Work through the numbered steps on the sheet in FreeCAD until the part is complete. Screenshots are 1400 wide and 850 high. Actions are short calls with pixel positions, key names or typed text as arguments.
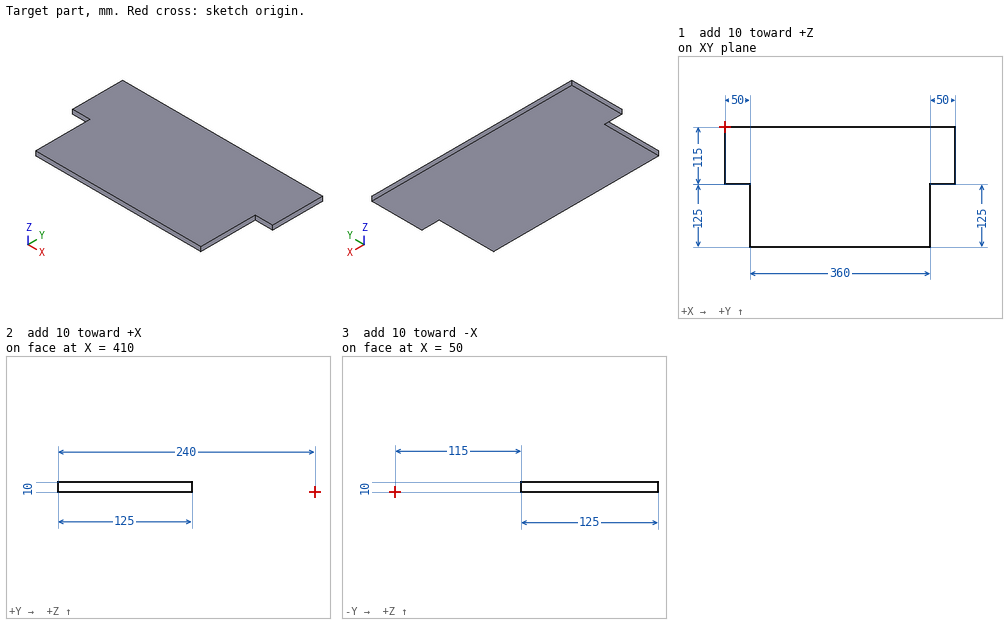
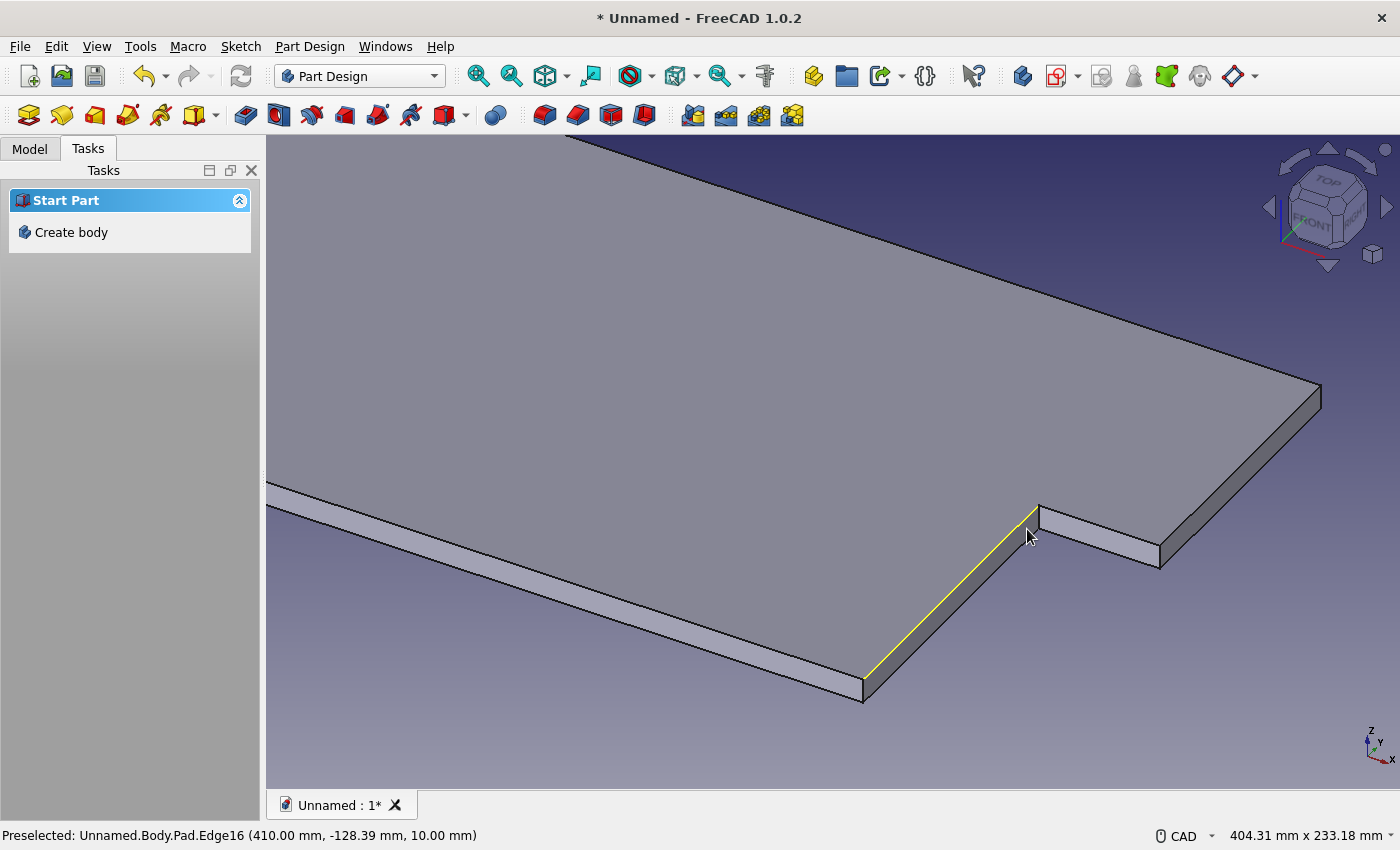
click(479, 76)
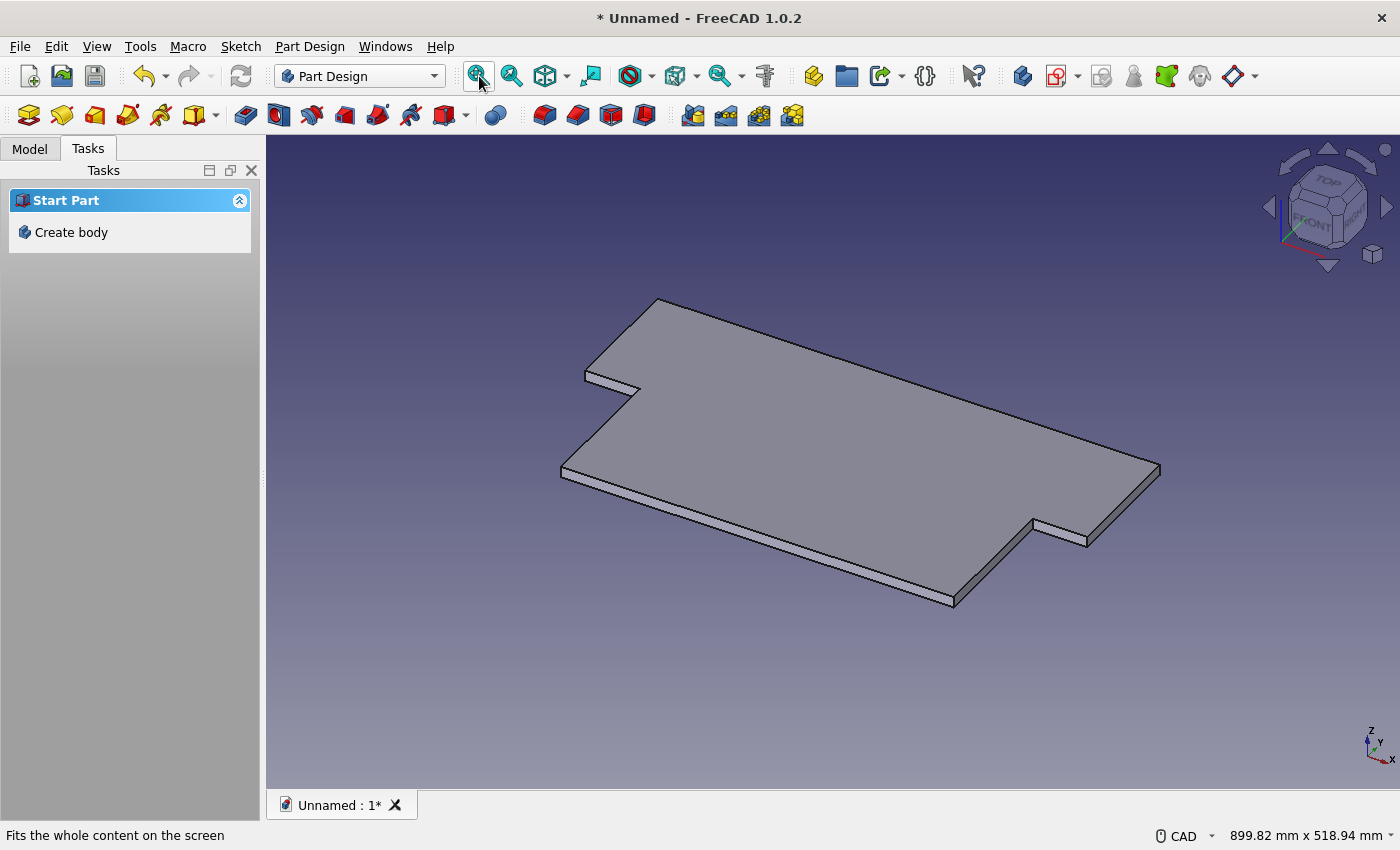
key(0)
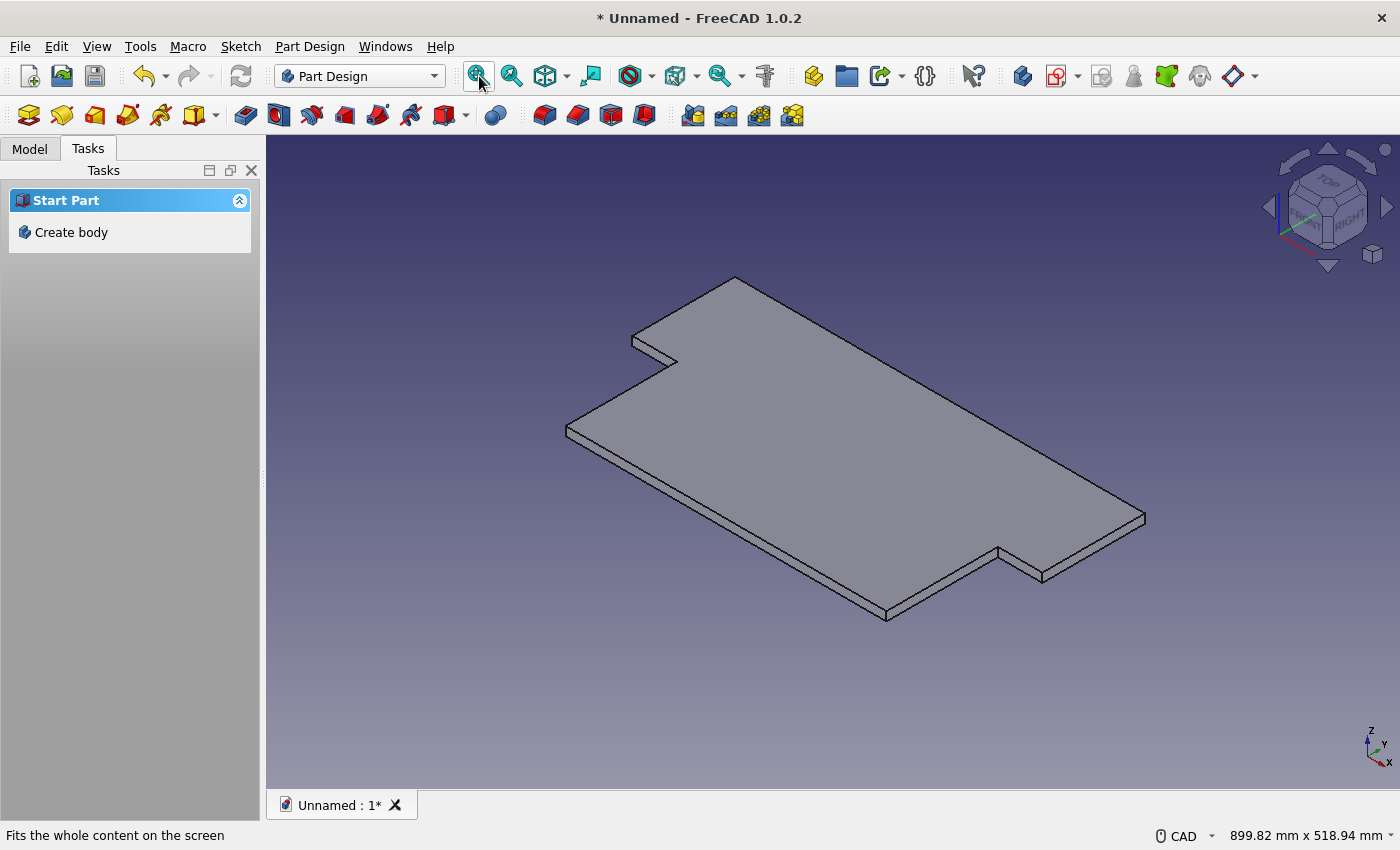
scroll(990, 556, up, 4)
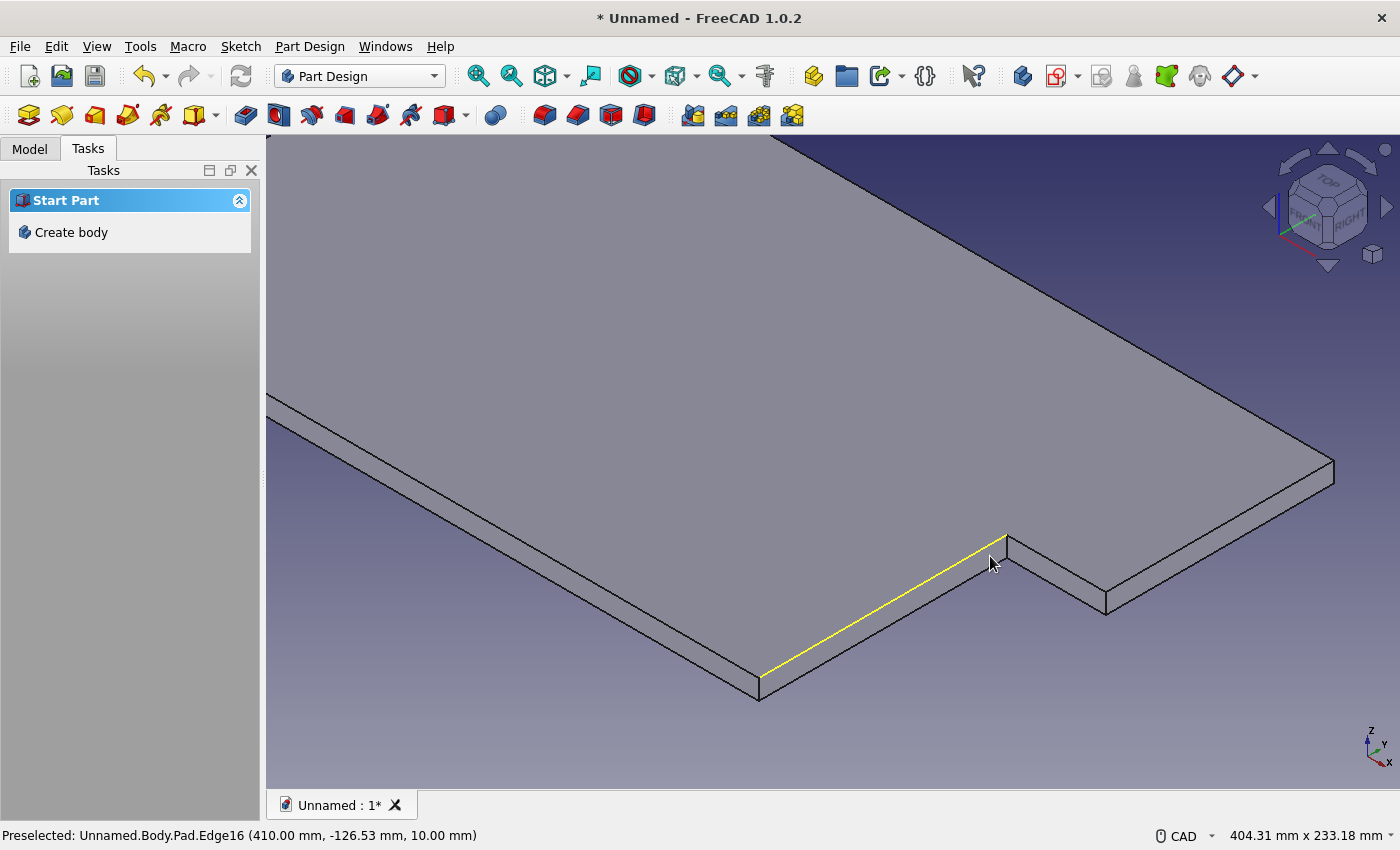
click(989, 556)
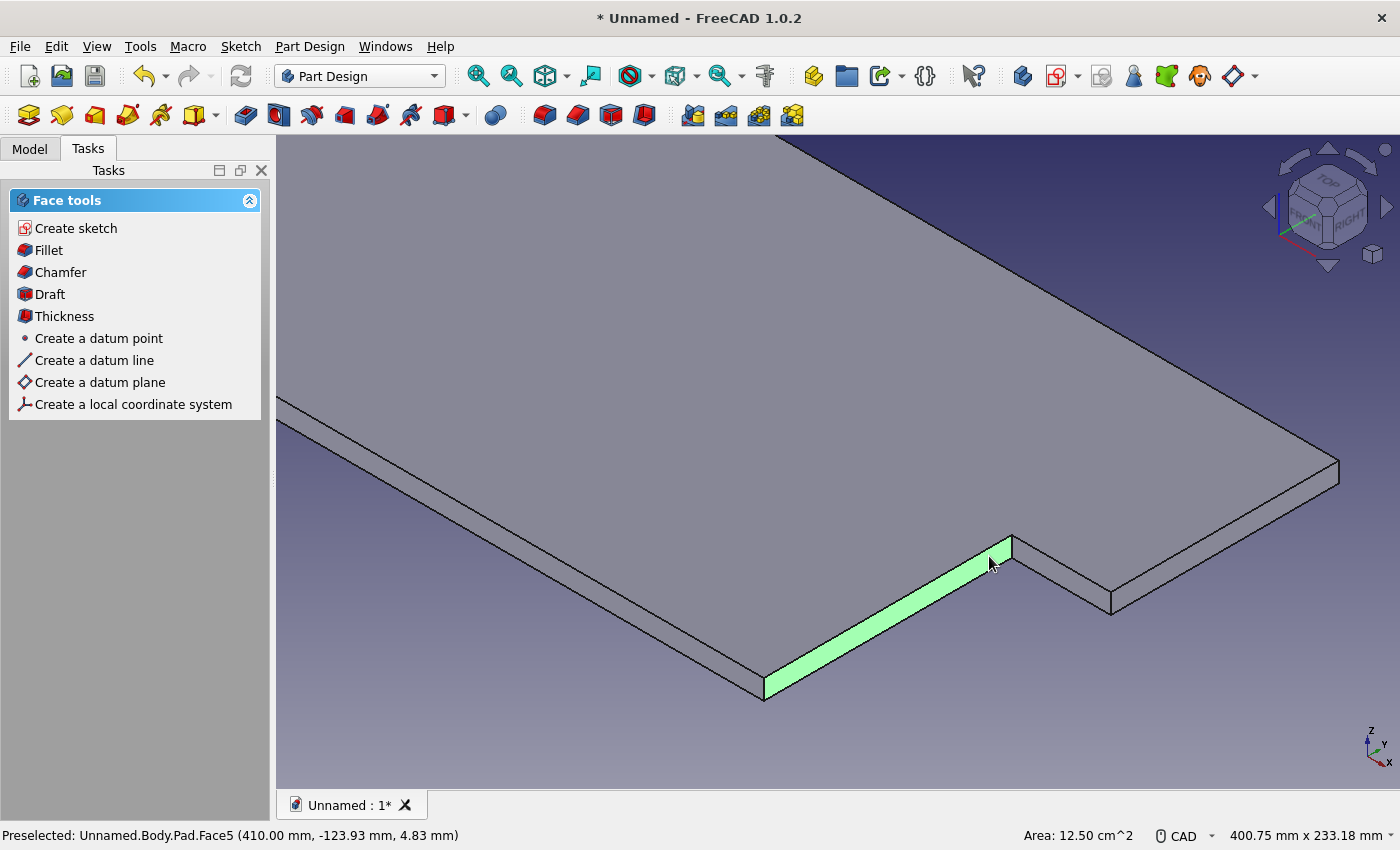
click(1056, 76)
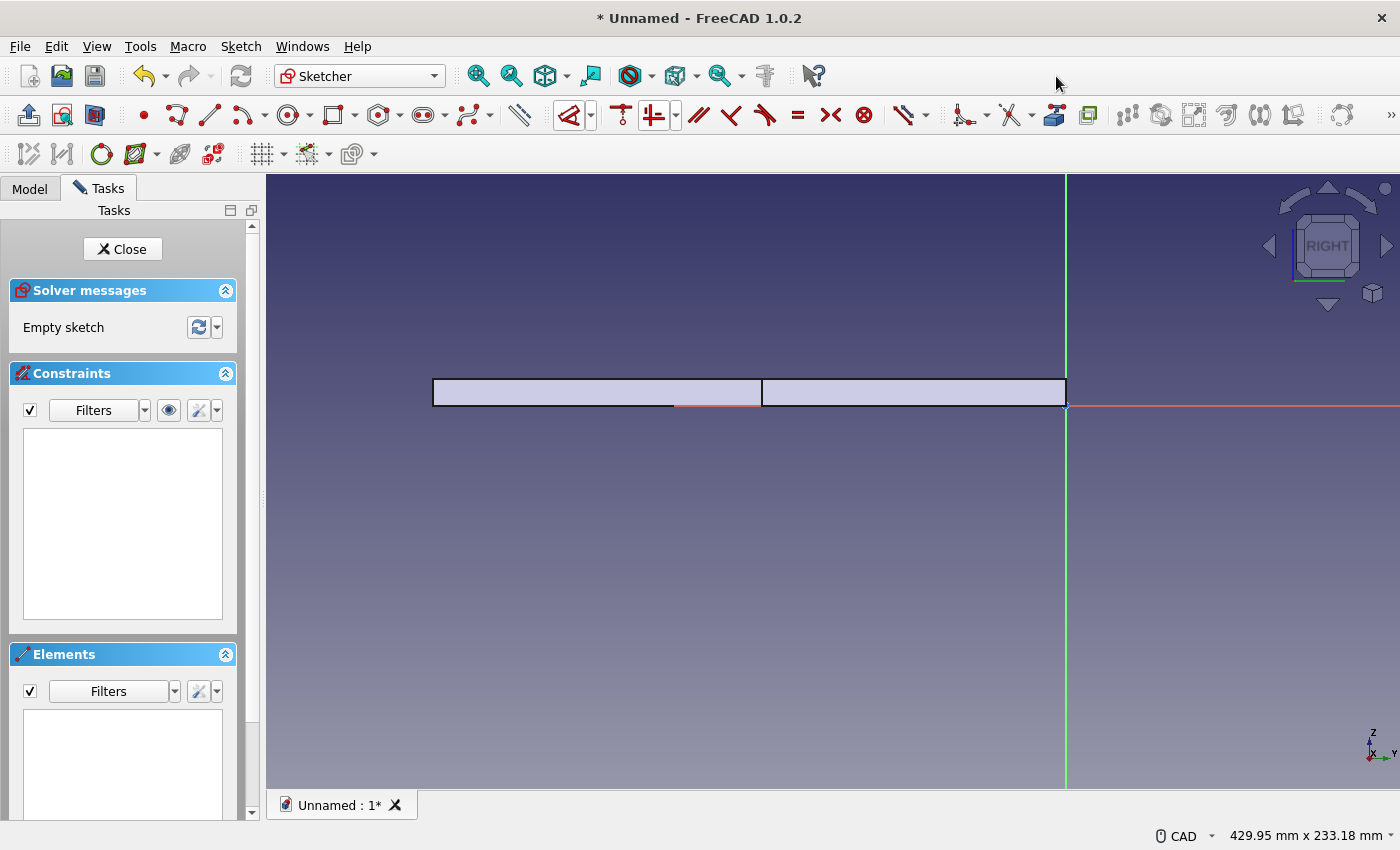
click(332, 116)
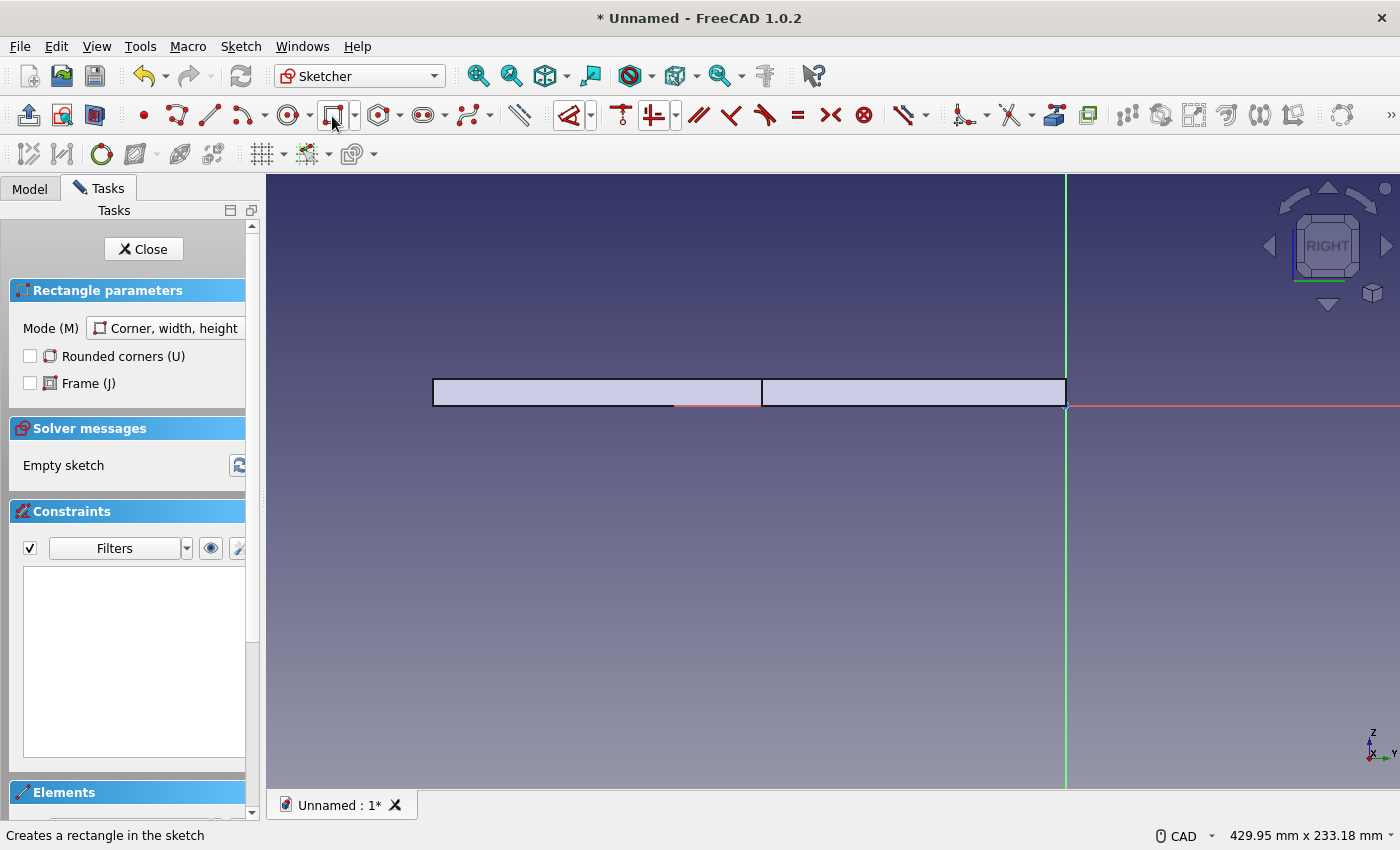
click(433, 379)
click(762, 406)
key(Escape)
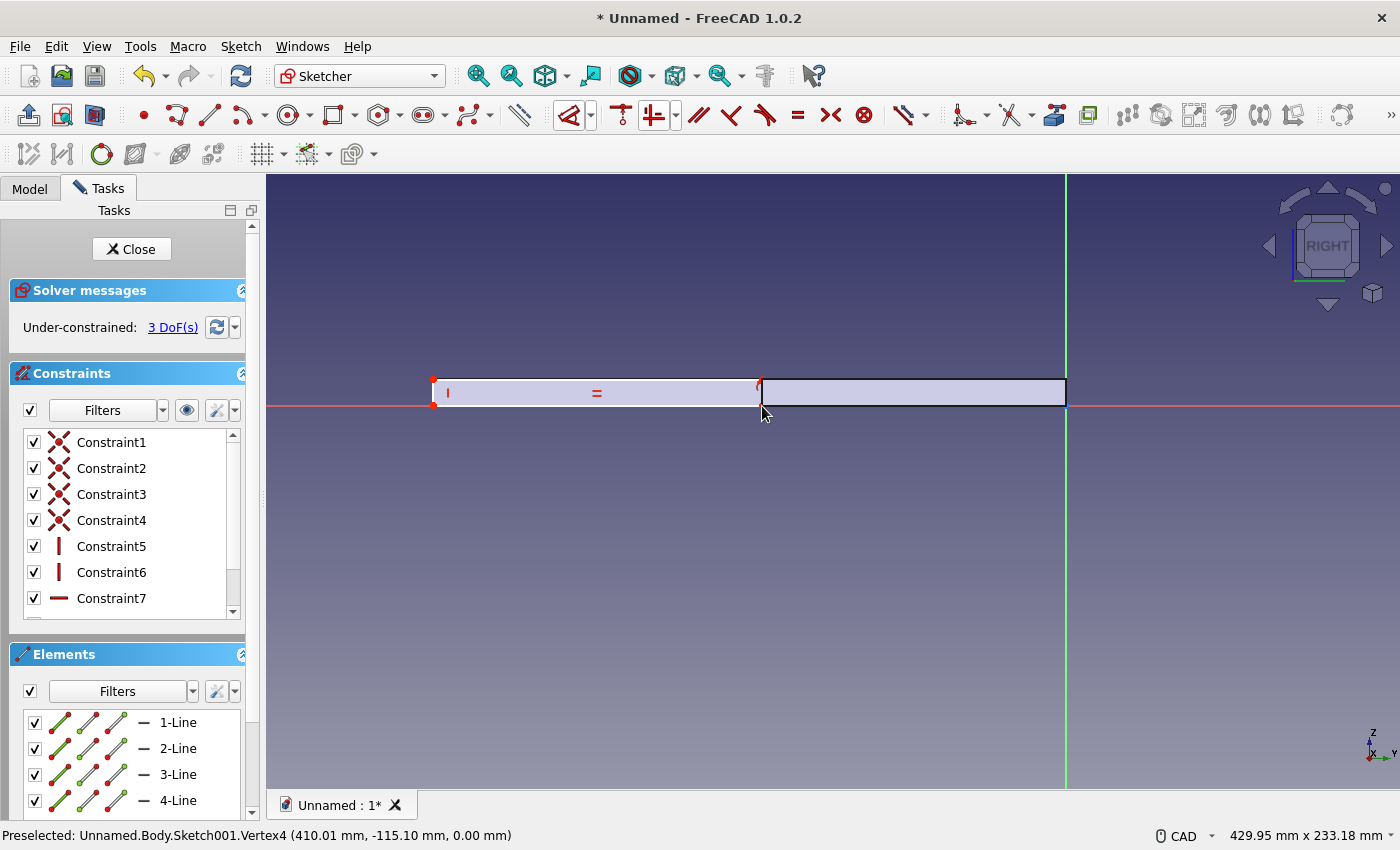
scroll(433, 390, up, 3)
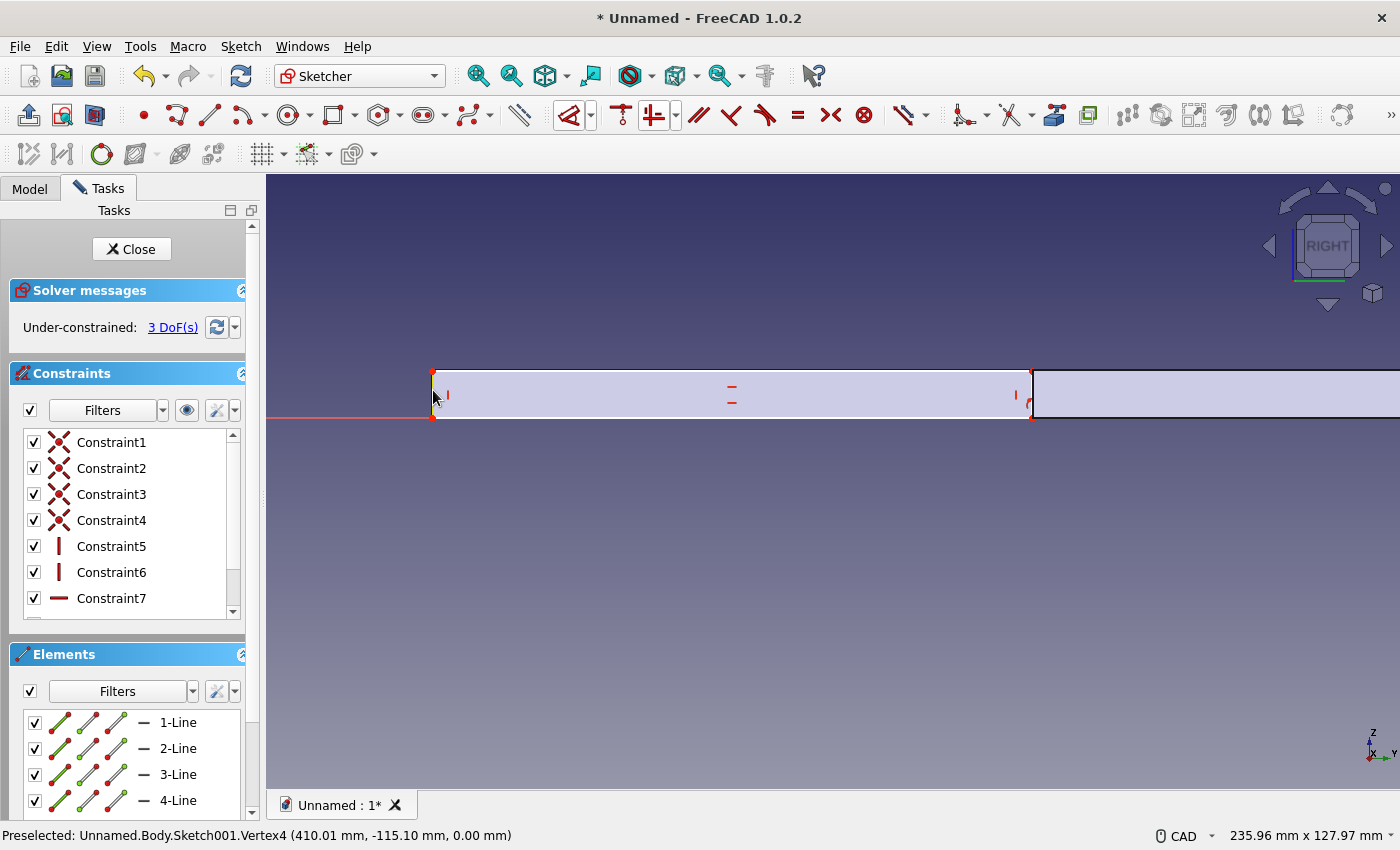
click(433, 390)